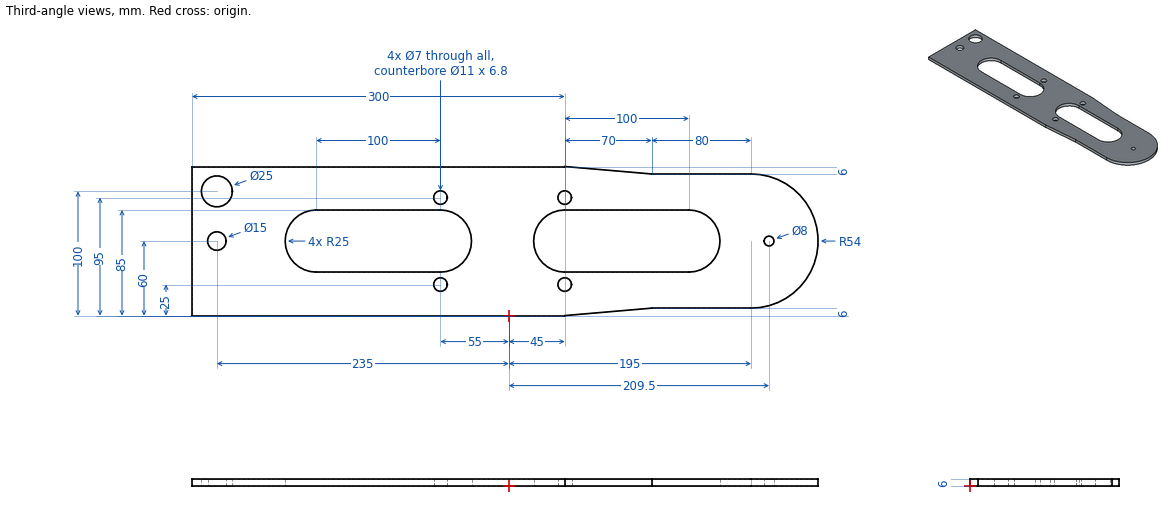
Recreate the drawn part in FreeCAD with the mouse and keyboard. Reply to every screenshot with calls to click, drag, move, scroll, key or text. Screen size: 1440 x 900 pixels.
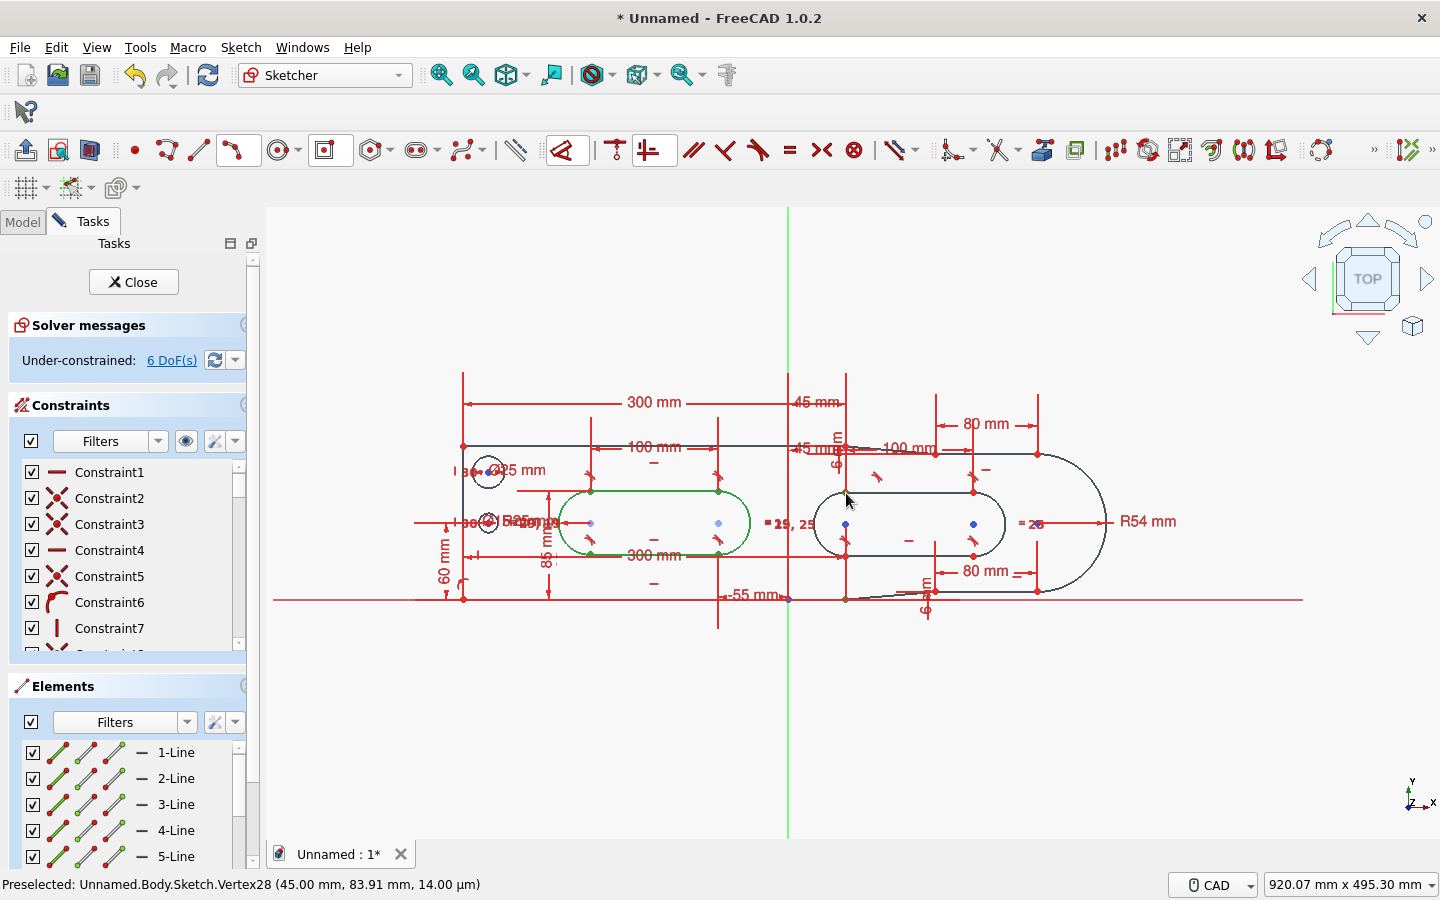
click(584, 150)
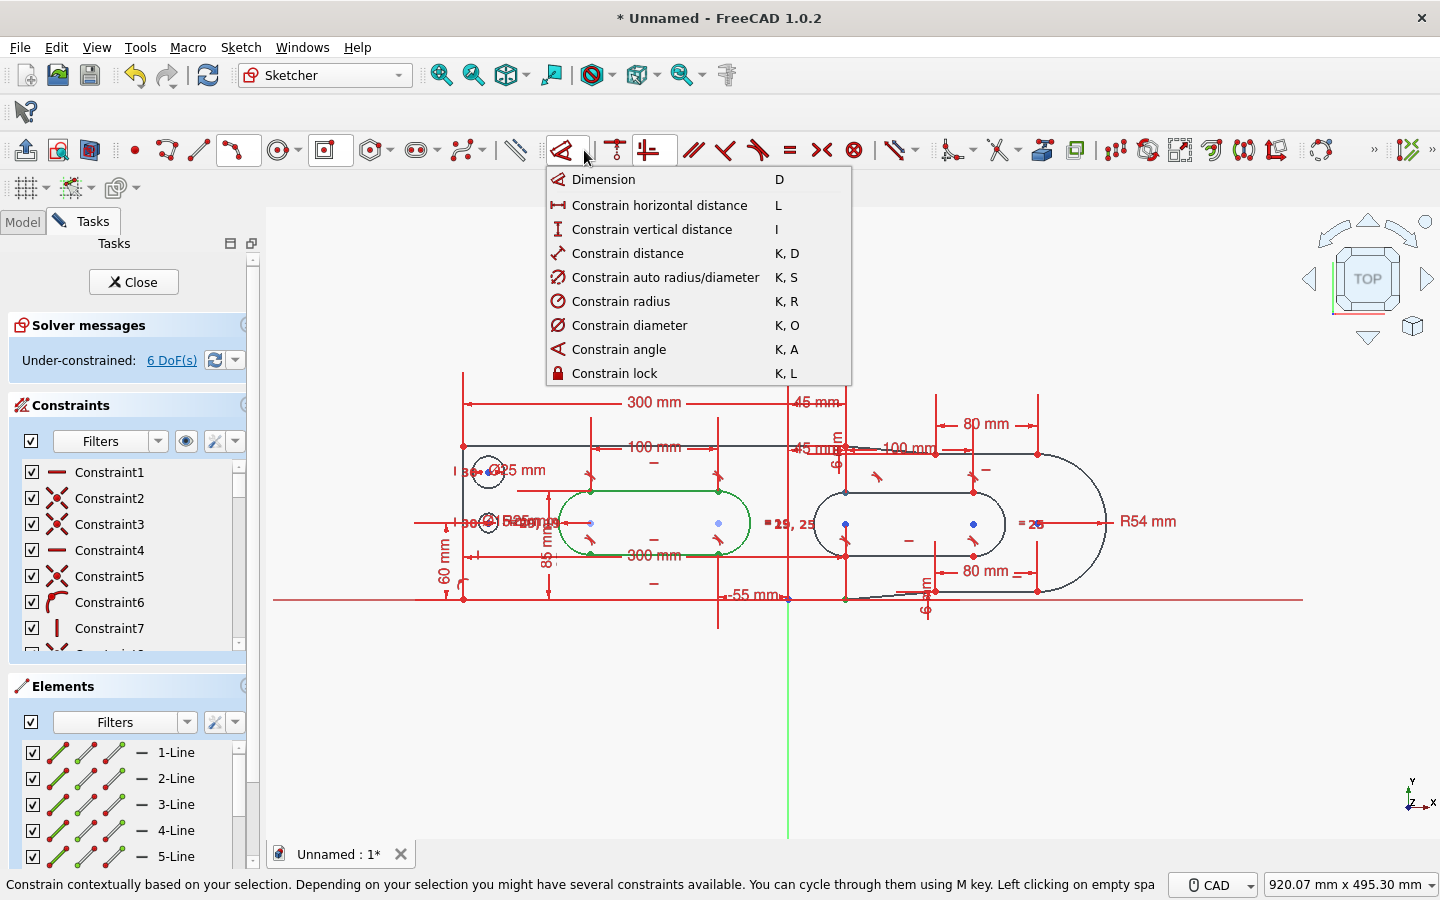
click(699, 229)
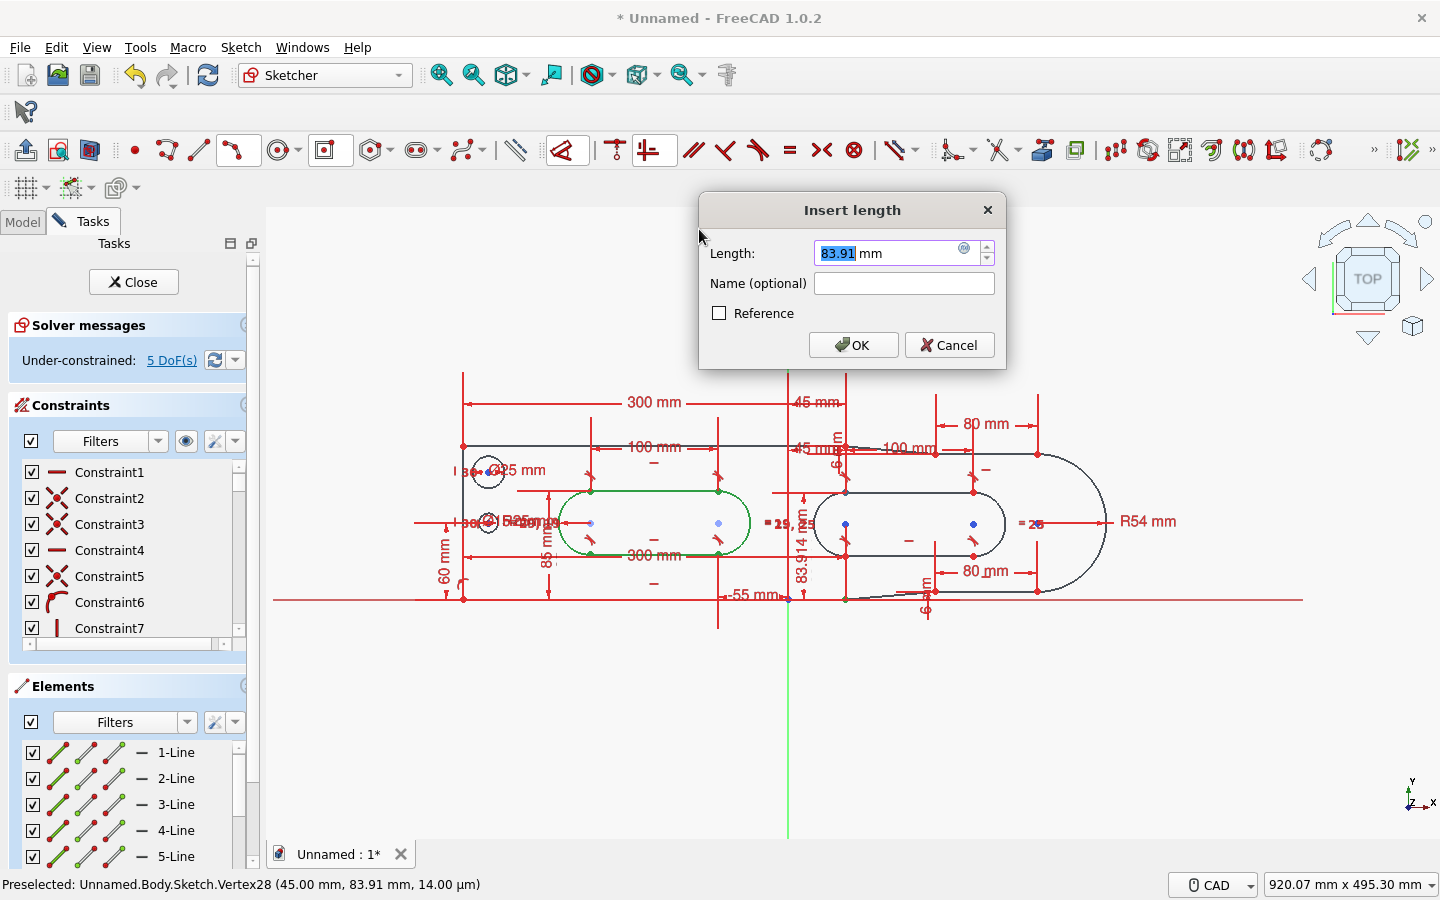
text(85)
key(Return)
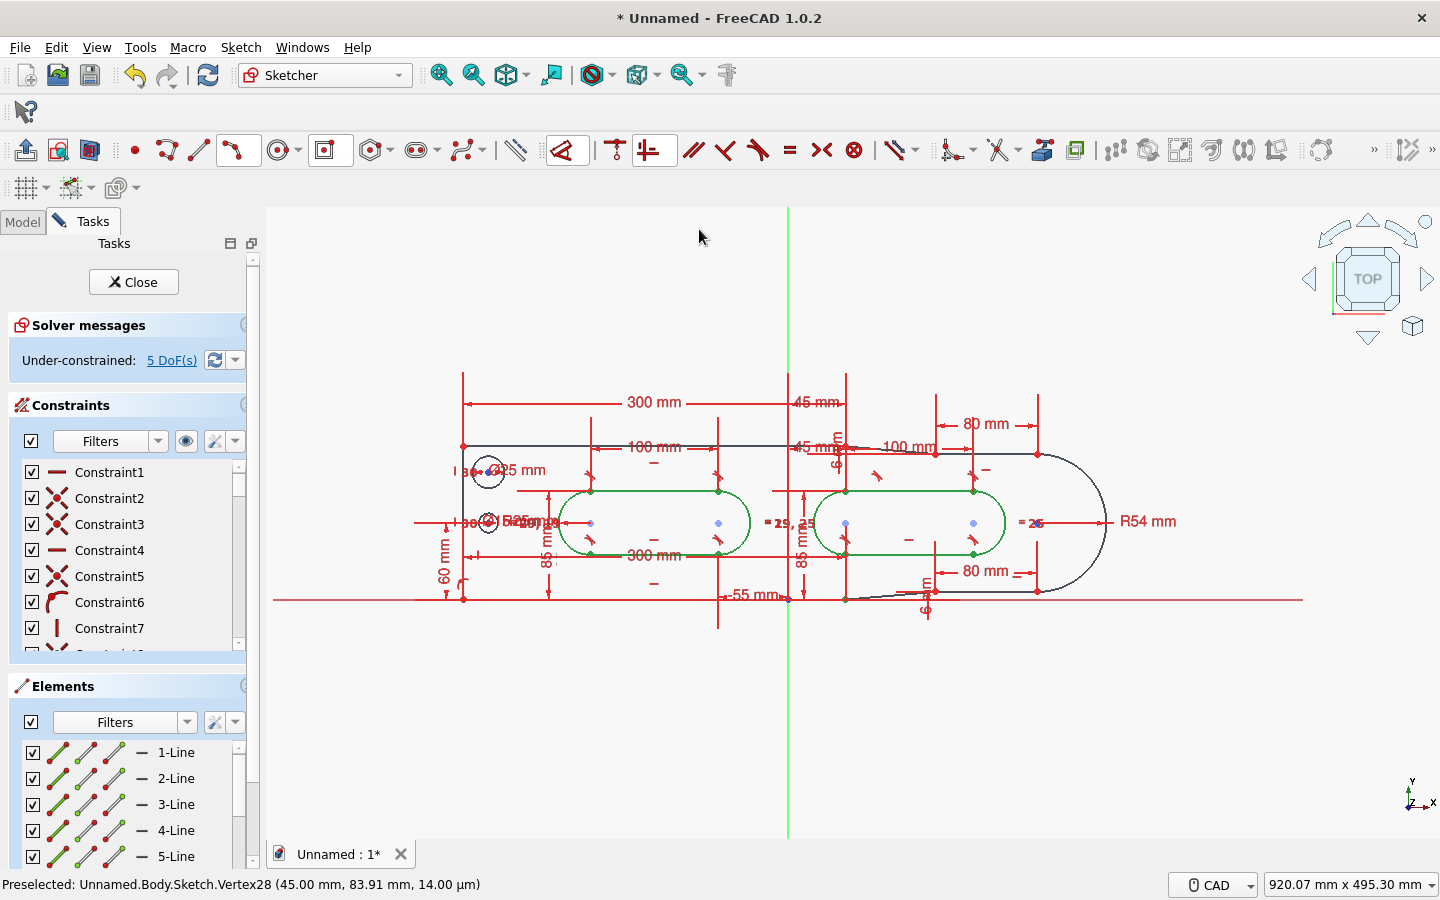
click(873, 449)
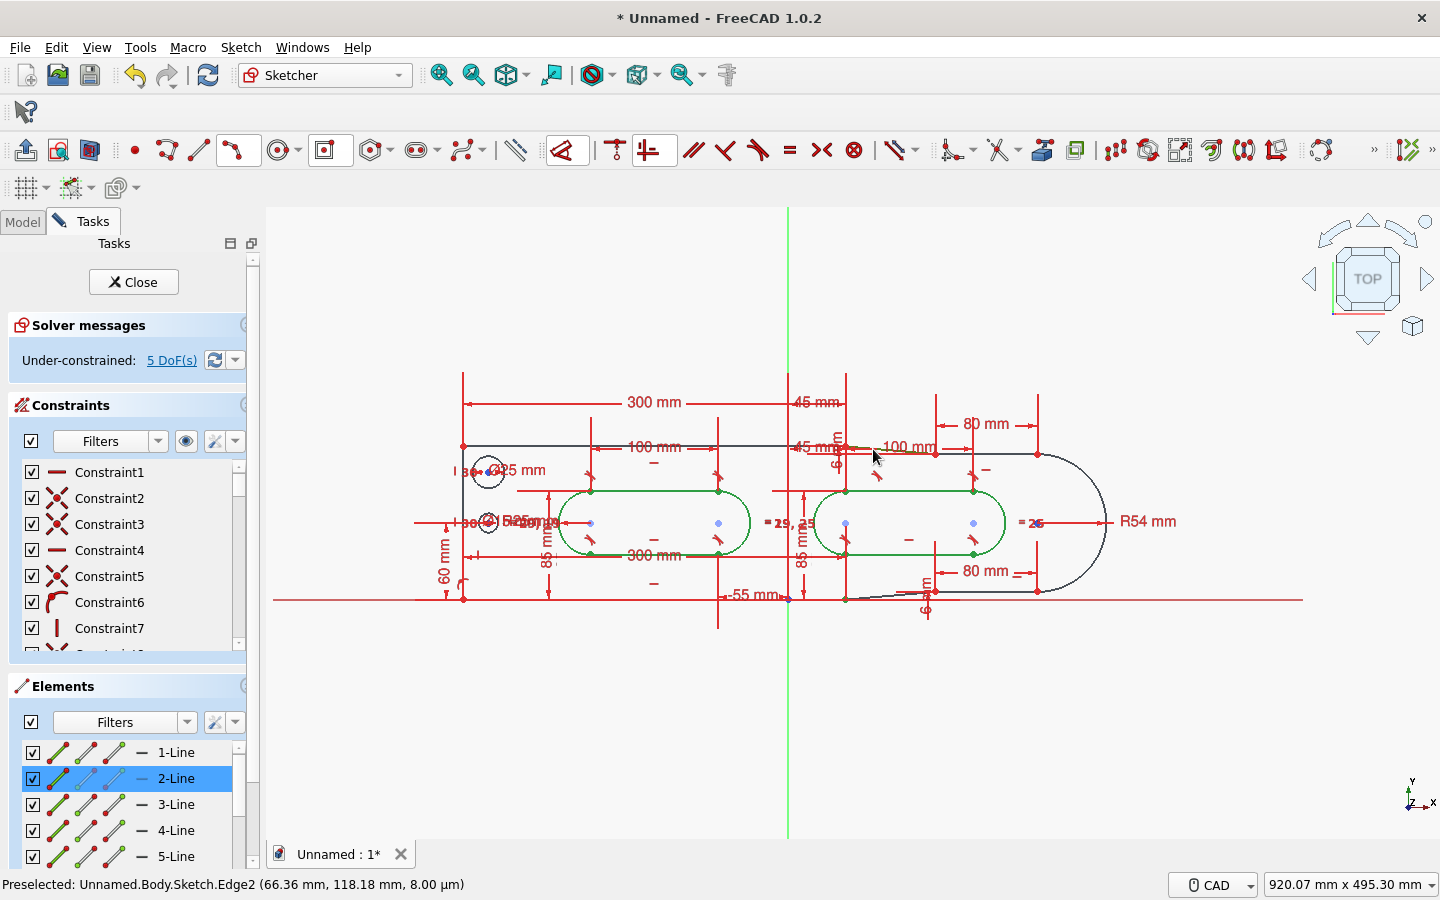
key(l)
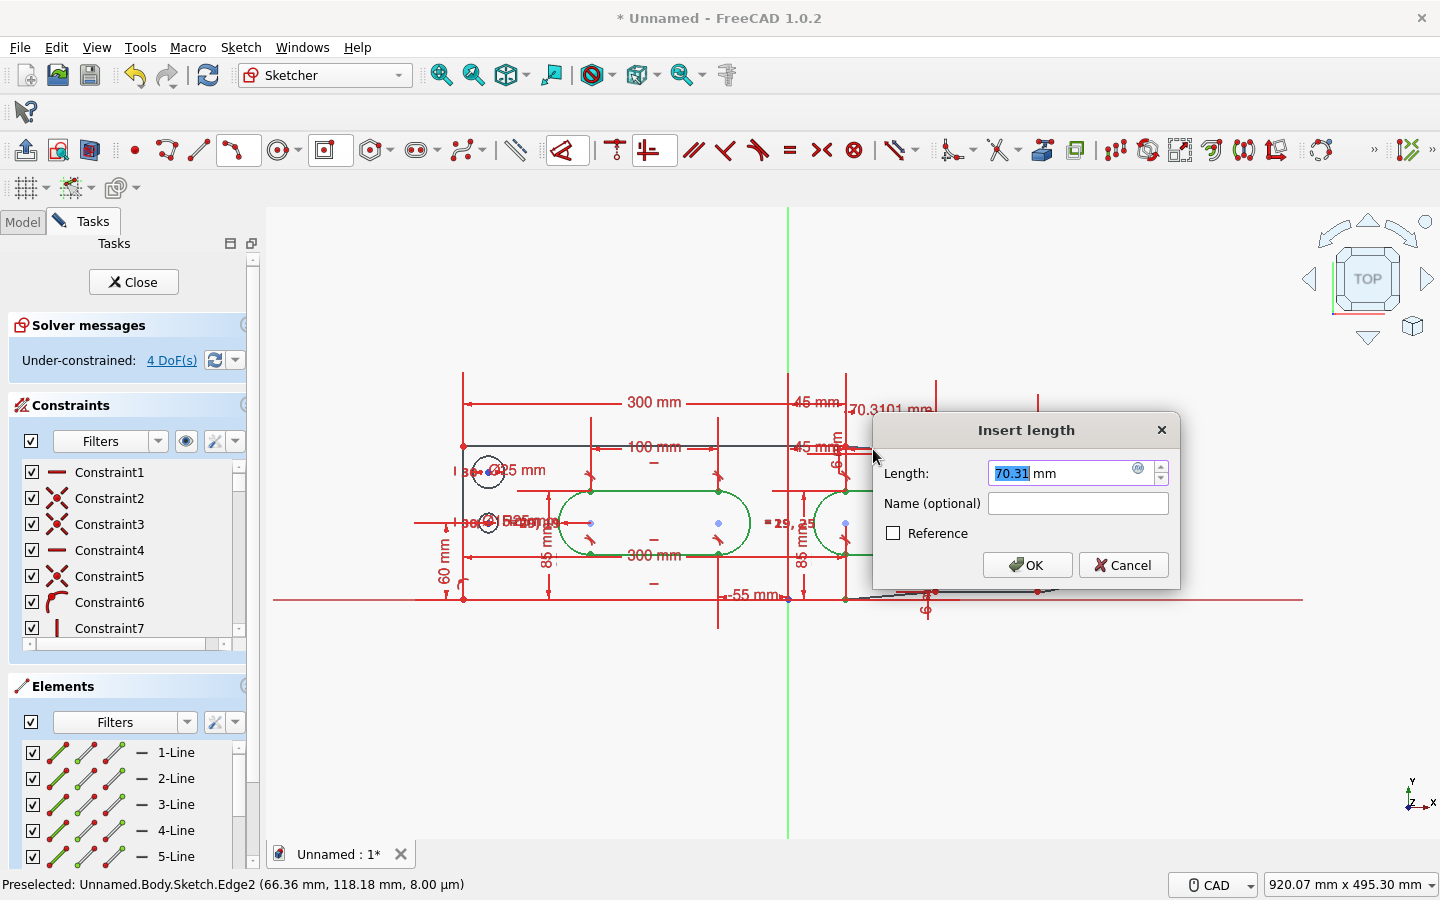
text(70)
key(Return)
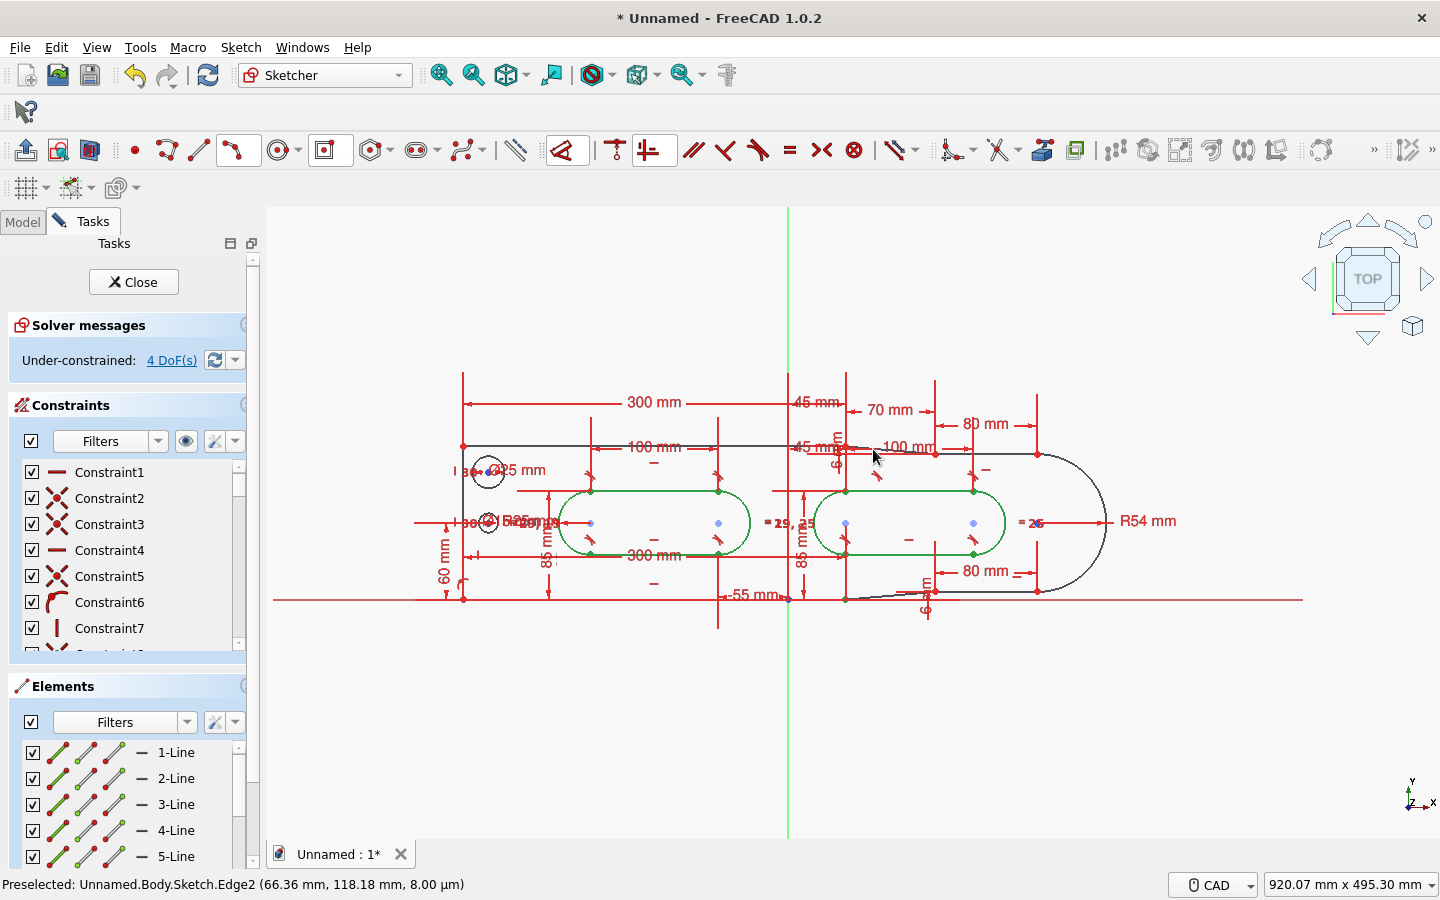
click(873, 597)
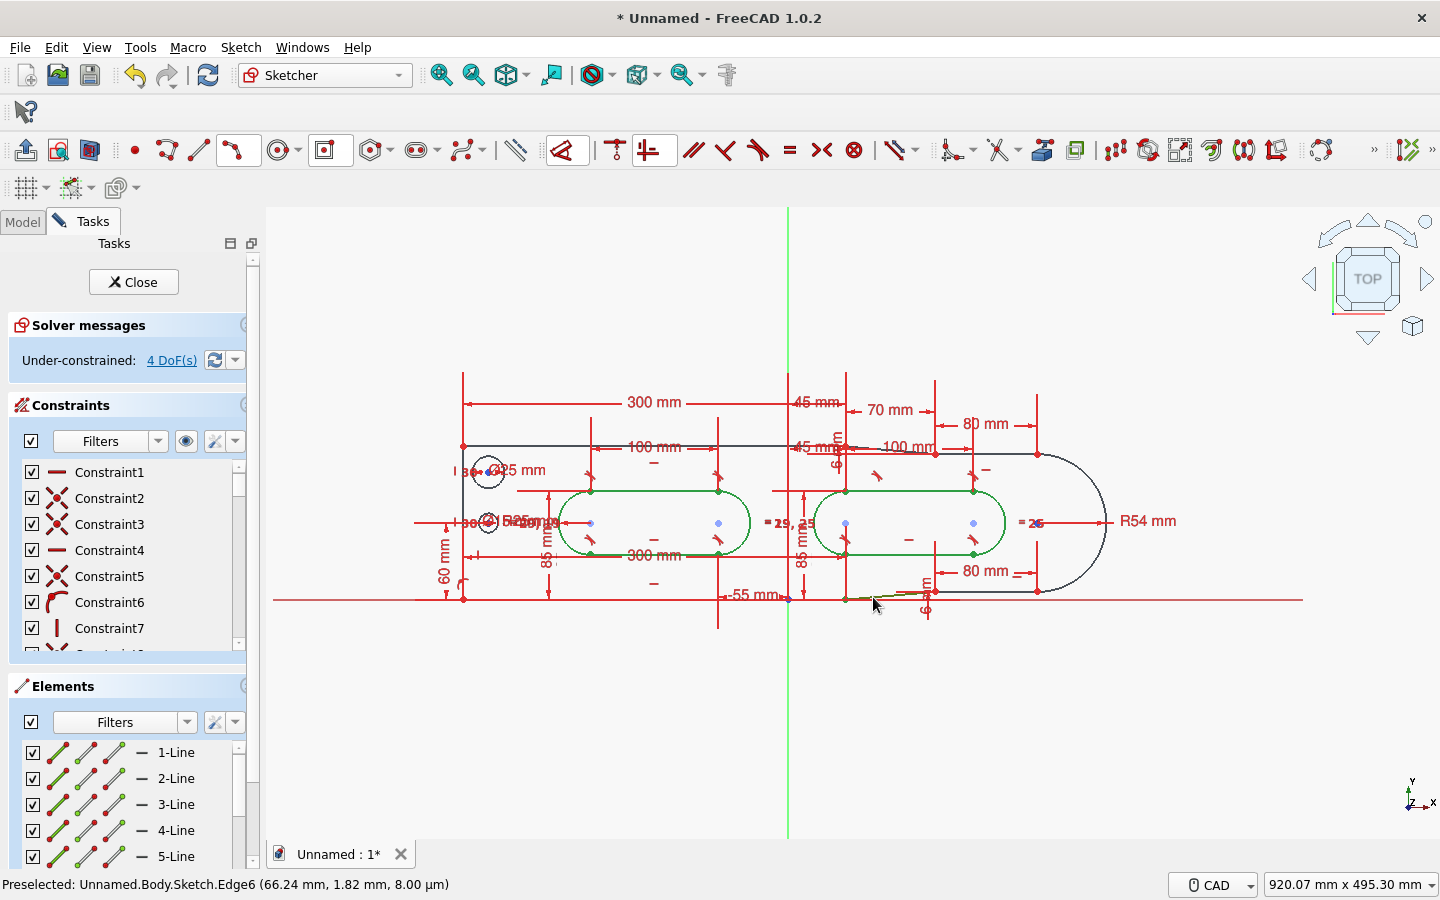
click(584, 150)